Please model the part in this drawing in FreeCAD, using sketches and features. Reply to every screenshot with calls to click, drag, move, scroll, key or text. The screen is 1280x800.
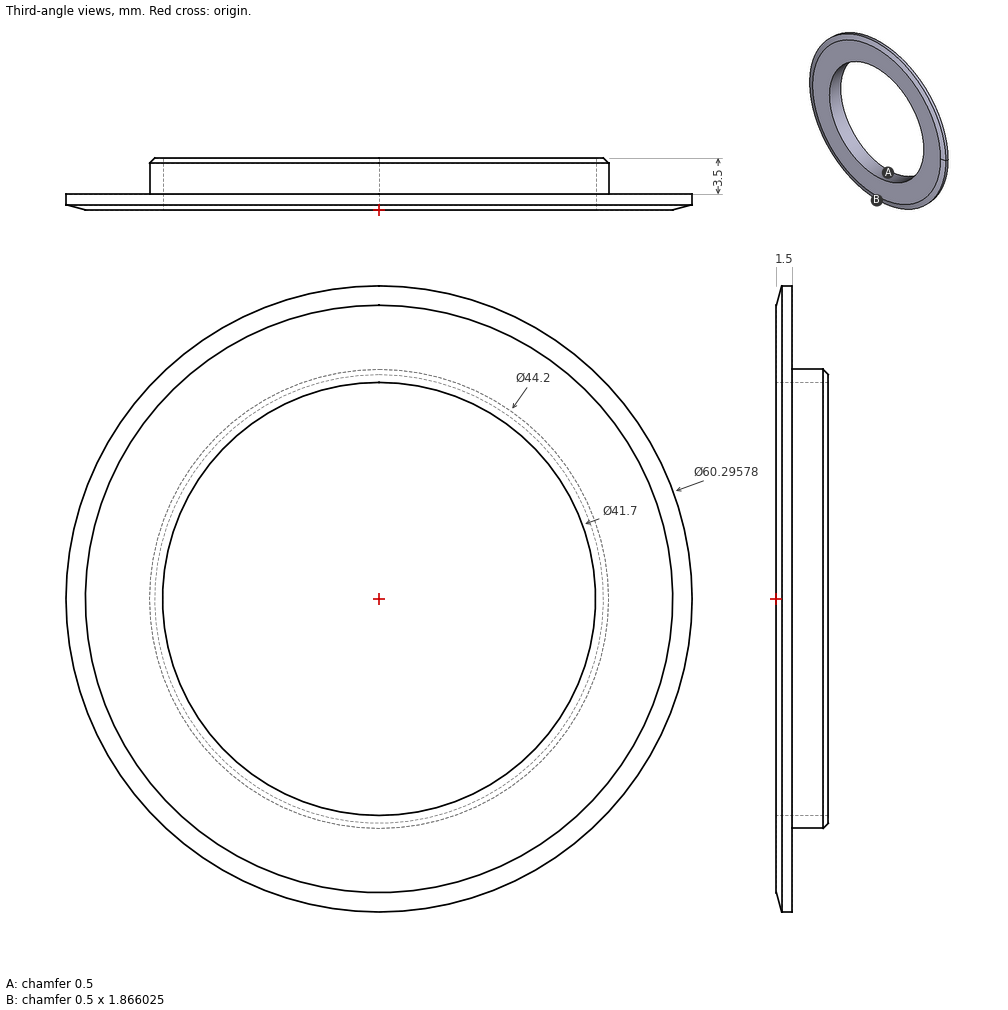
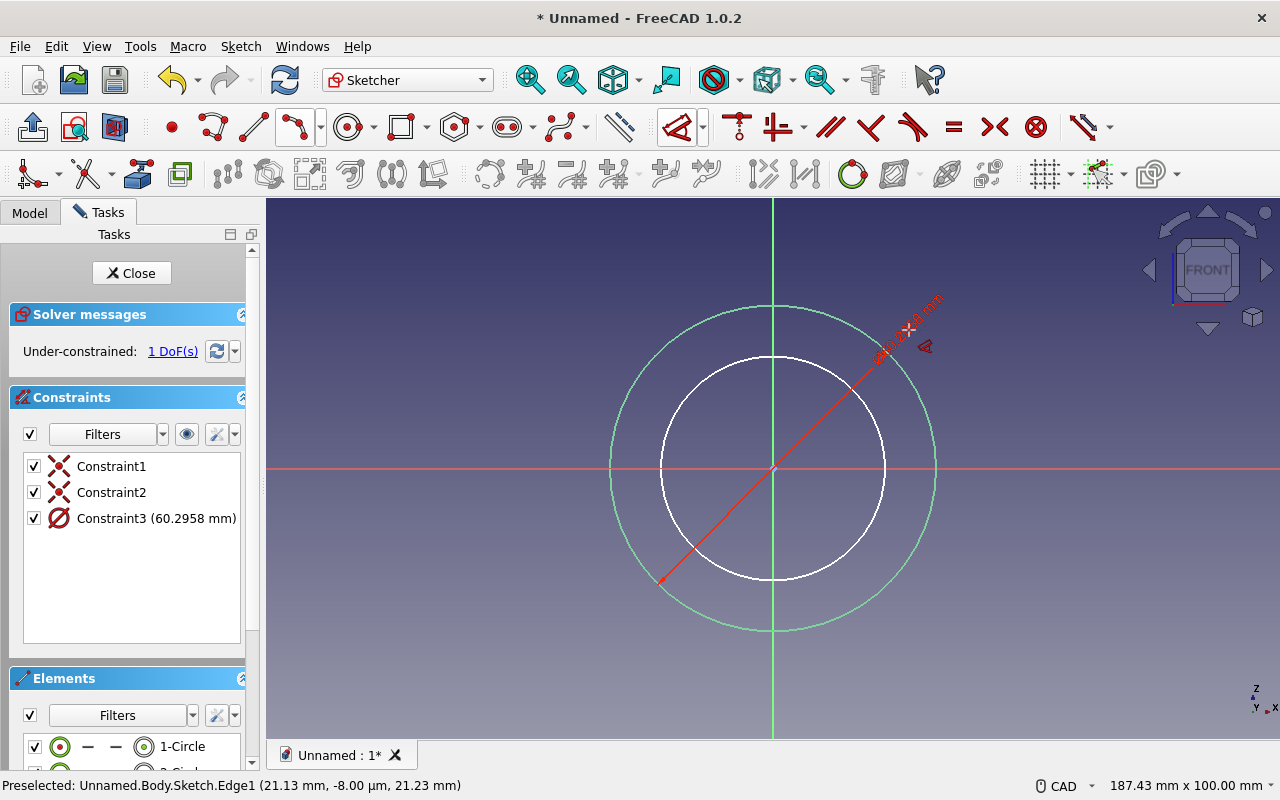
click(852, 389)
click(875, 366)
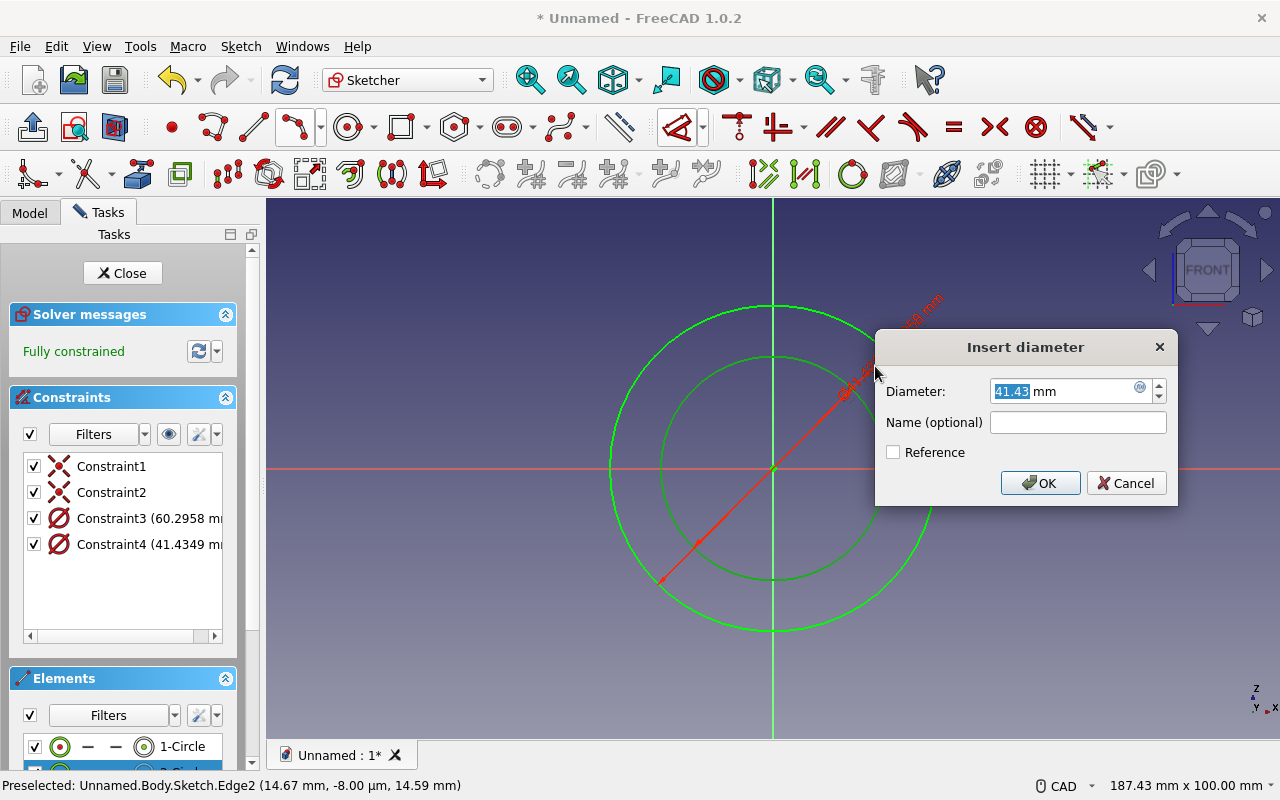
text(41.7)
key(Return)
key(Escape)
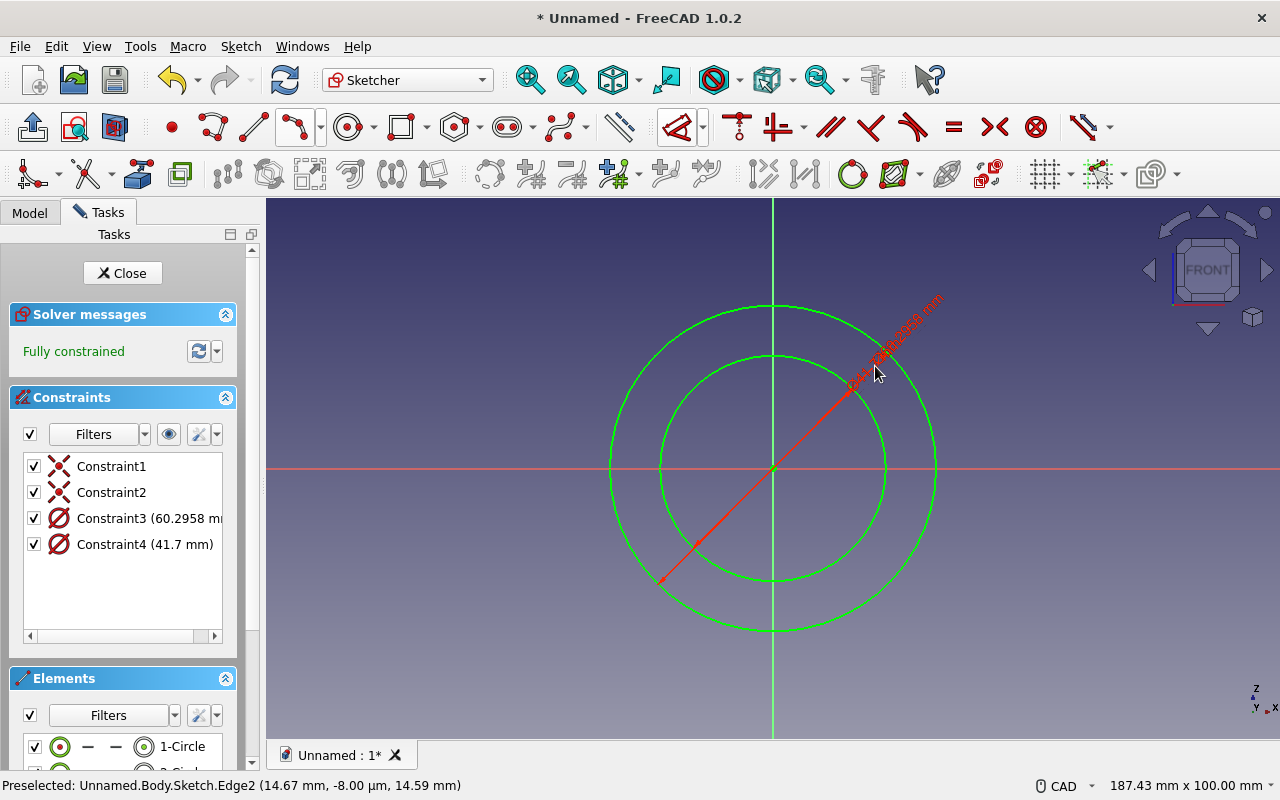
click(123, 273)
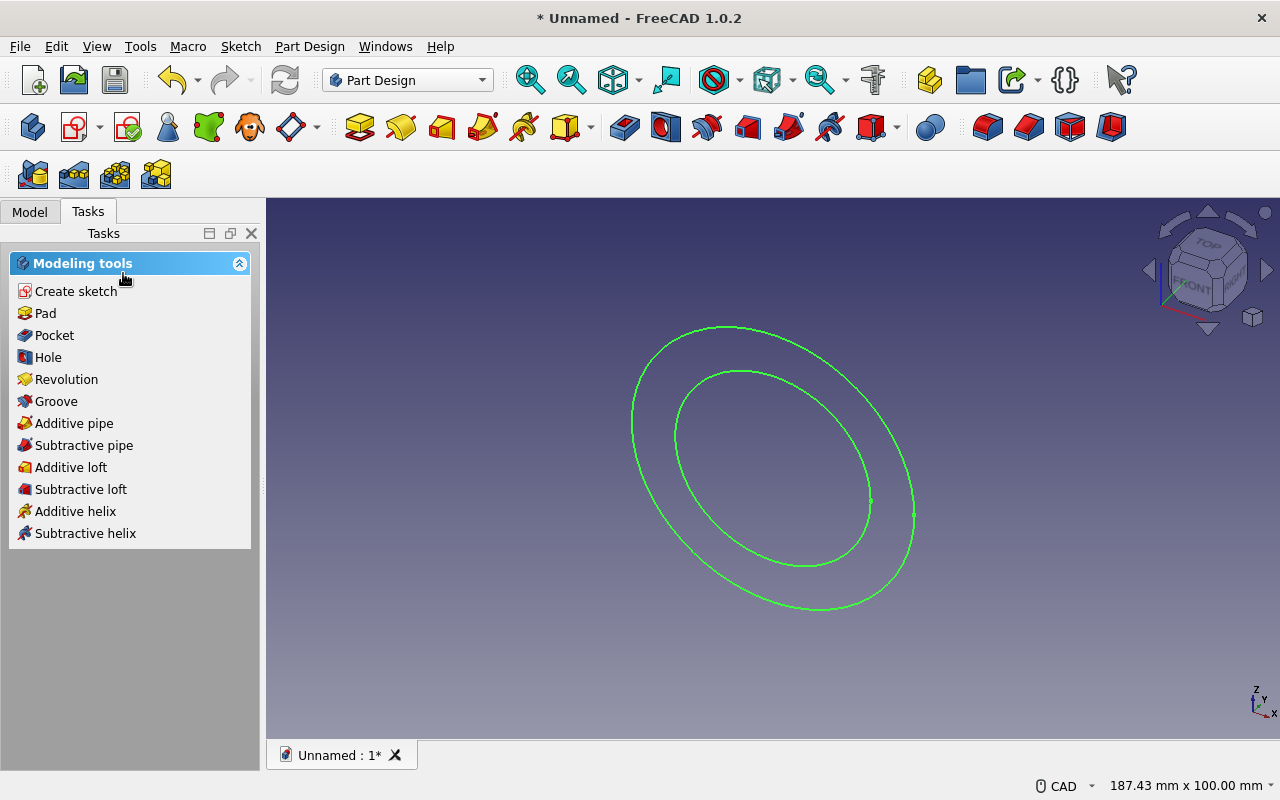
click(360, 128)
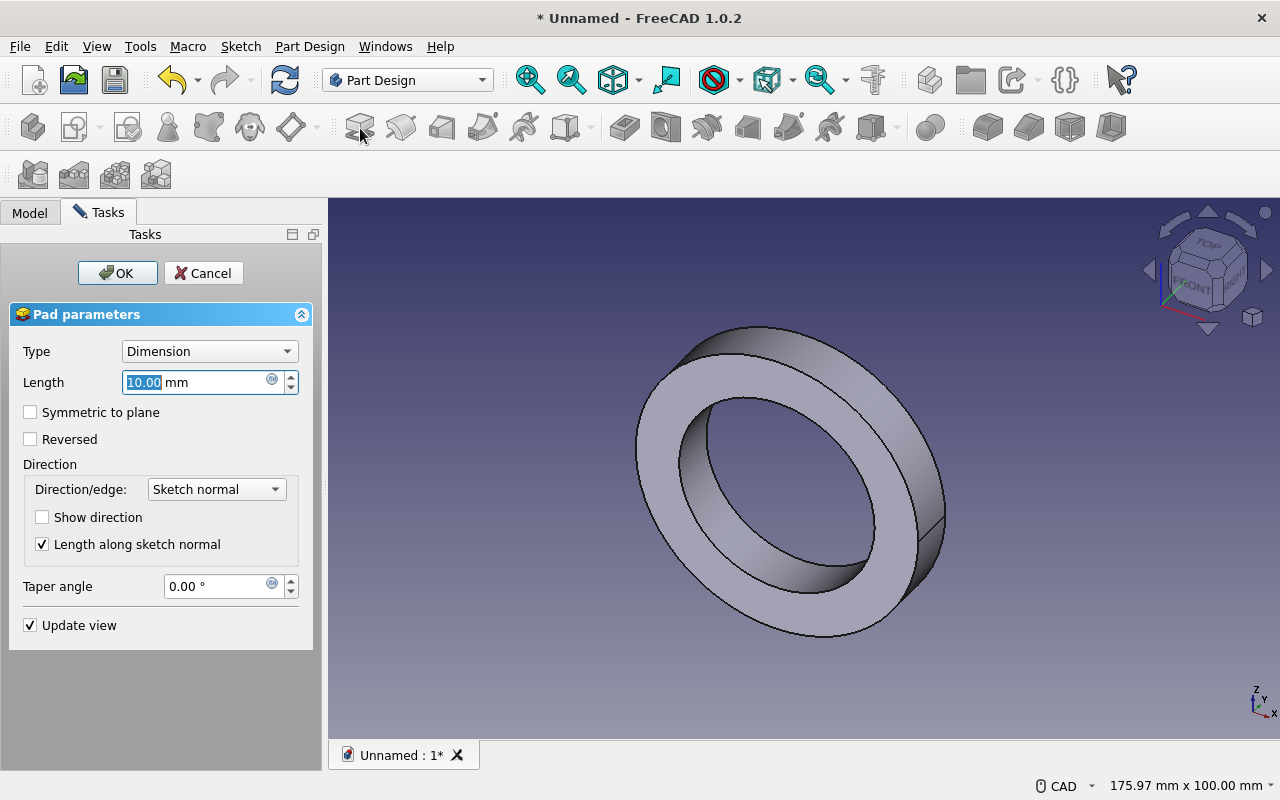
text(1.5)
key(Tab)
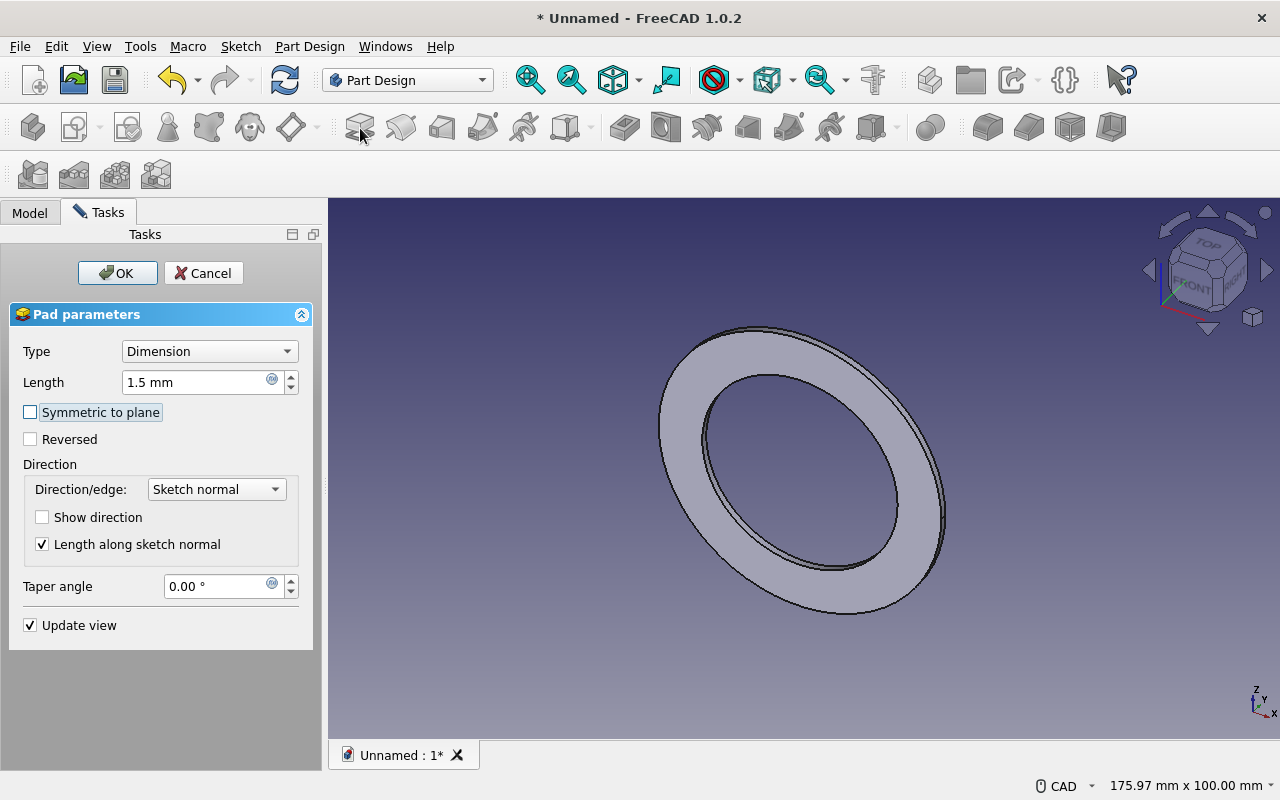
click(31, 439)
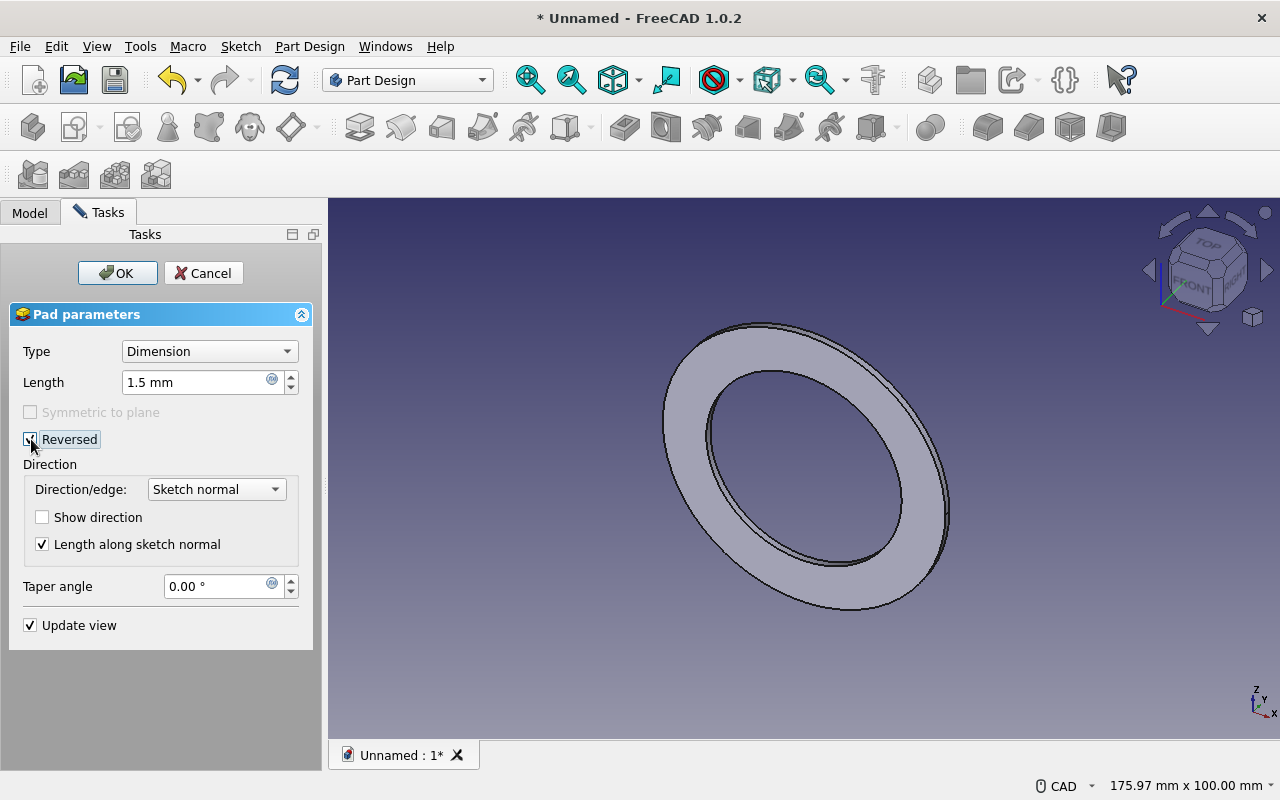
click(118, 273)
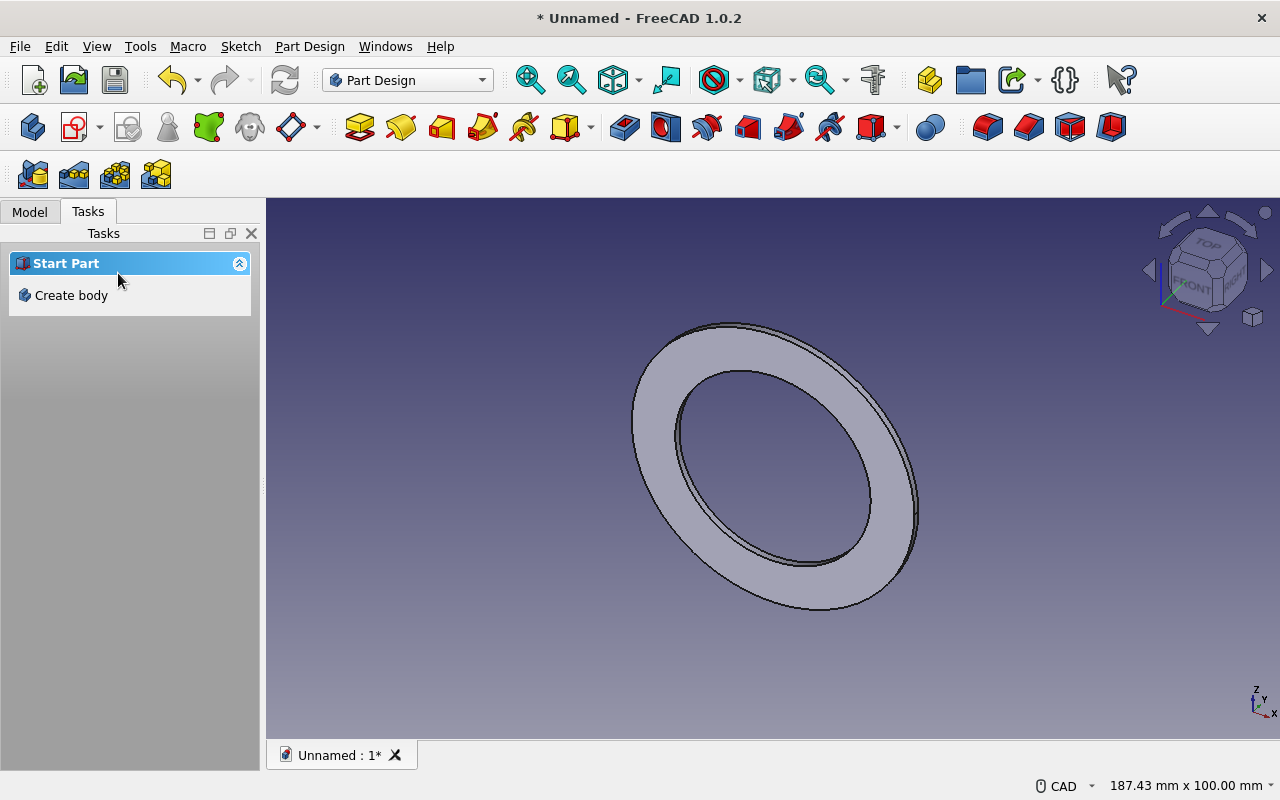
key(4)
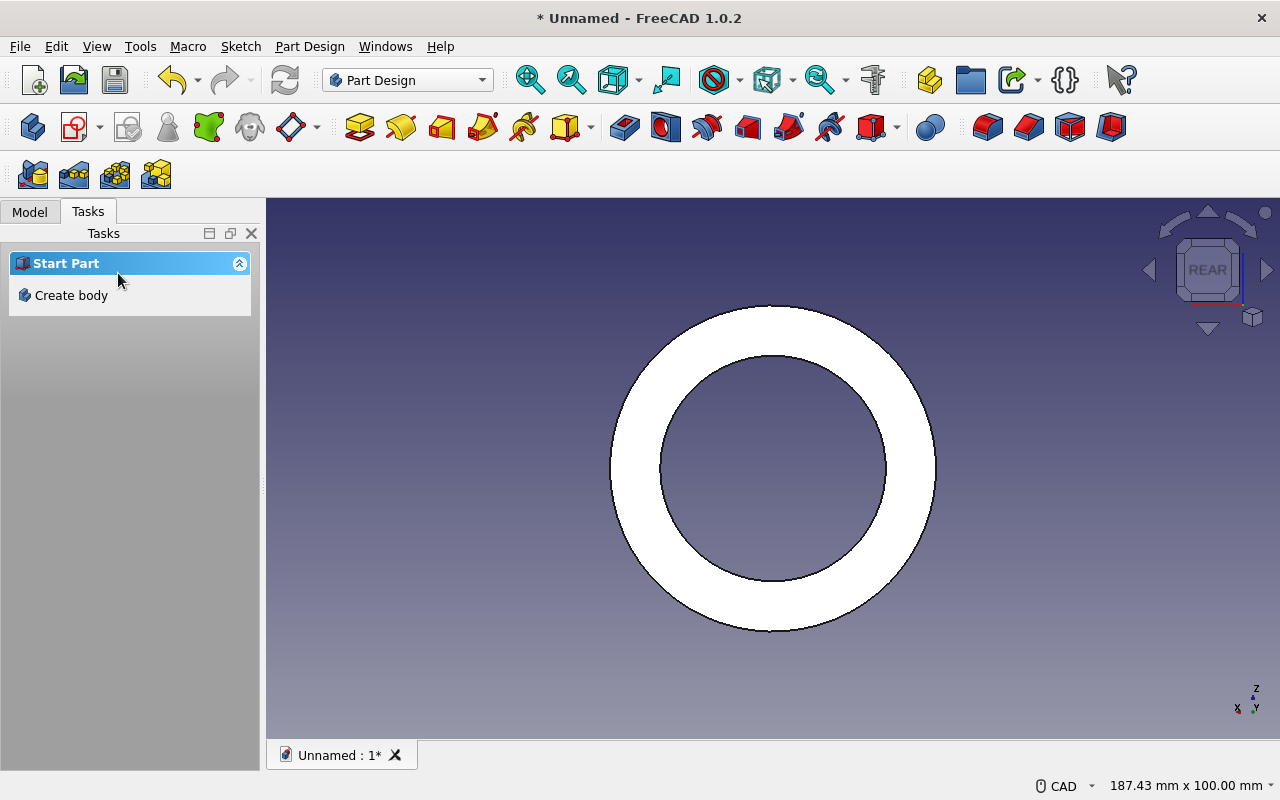
click(633, 467)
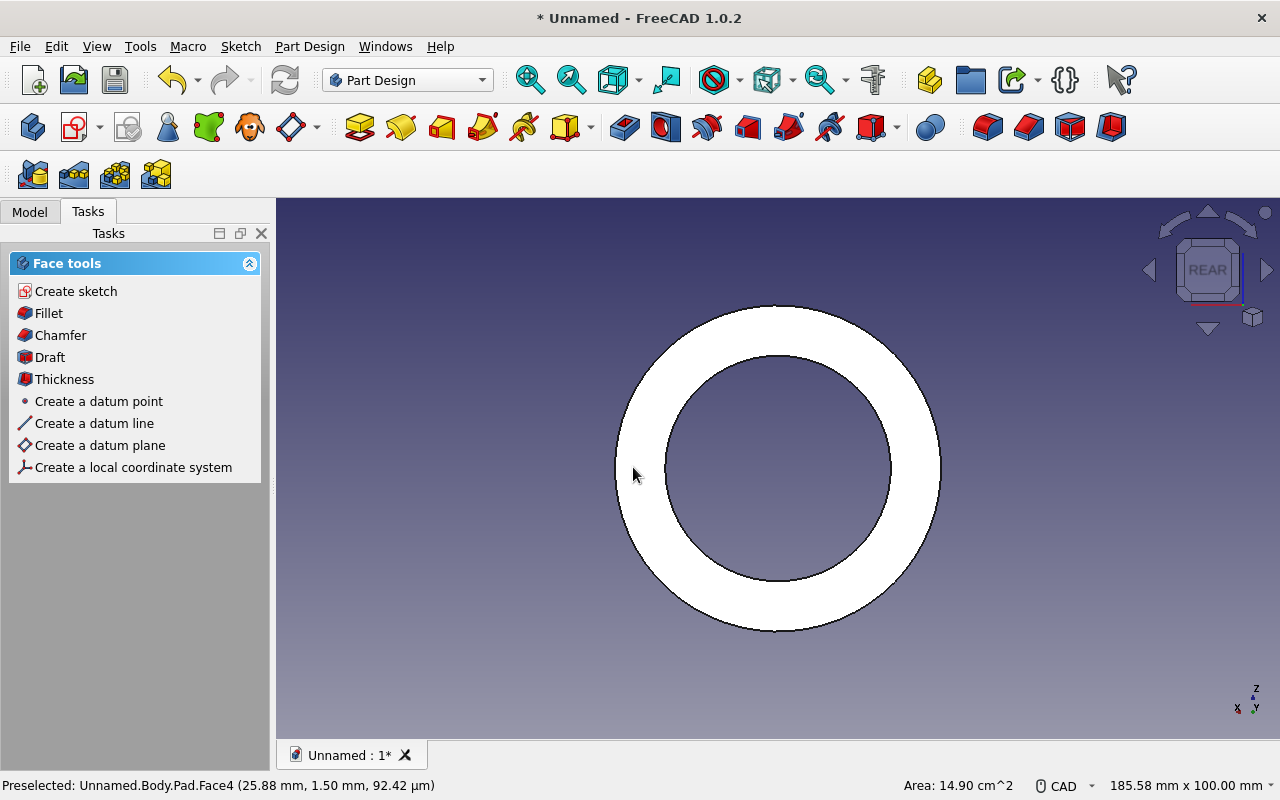
click(74, 128)